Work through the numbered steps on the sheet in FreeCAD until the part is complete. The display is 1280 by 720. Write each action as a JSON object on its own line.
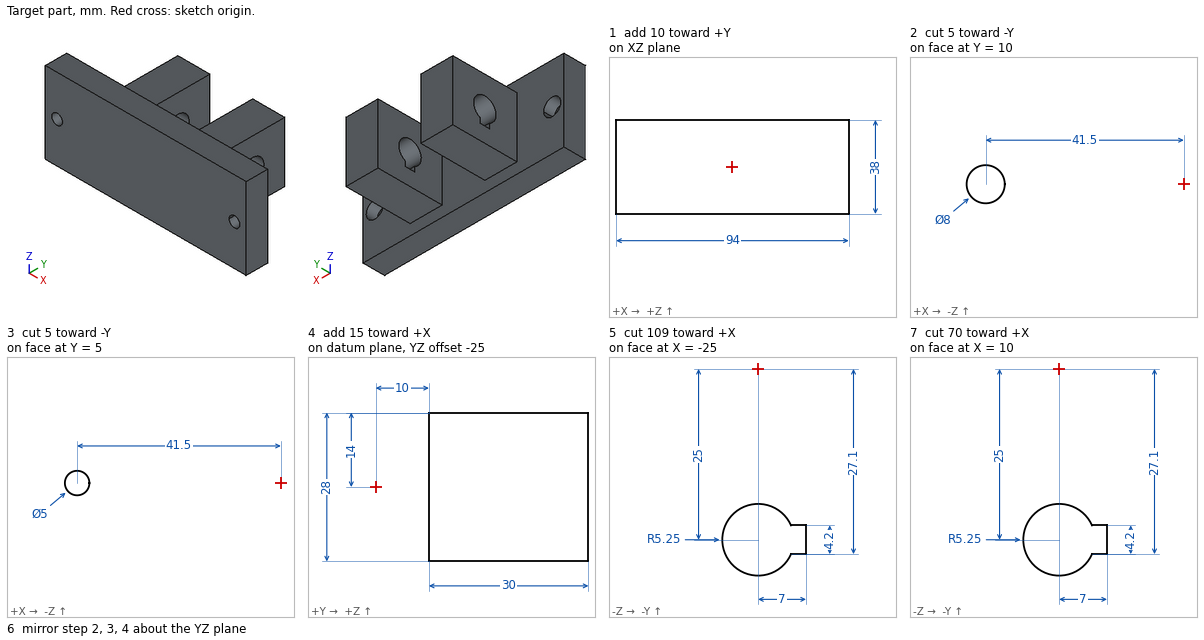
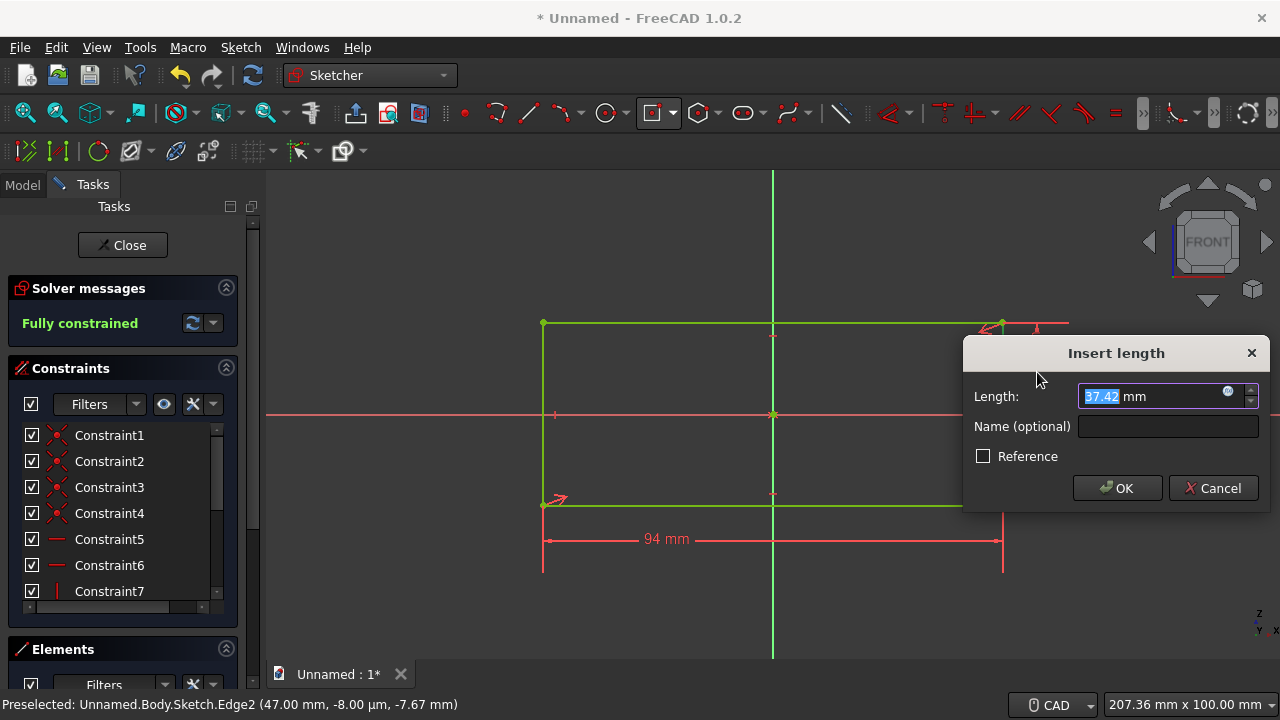
{"action": "type", "text": "38"}
{"action": "key", "text": "Return"}
{"action": "key", "text": "Escape"}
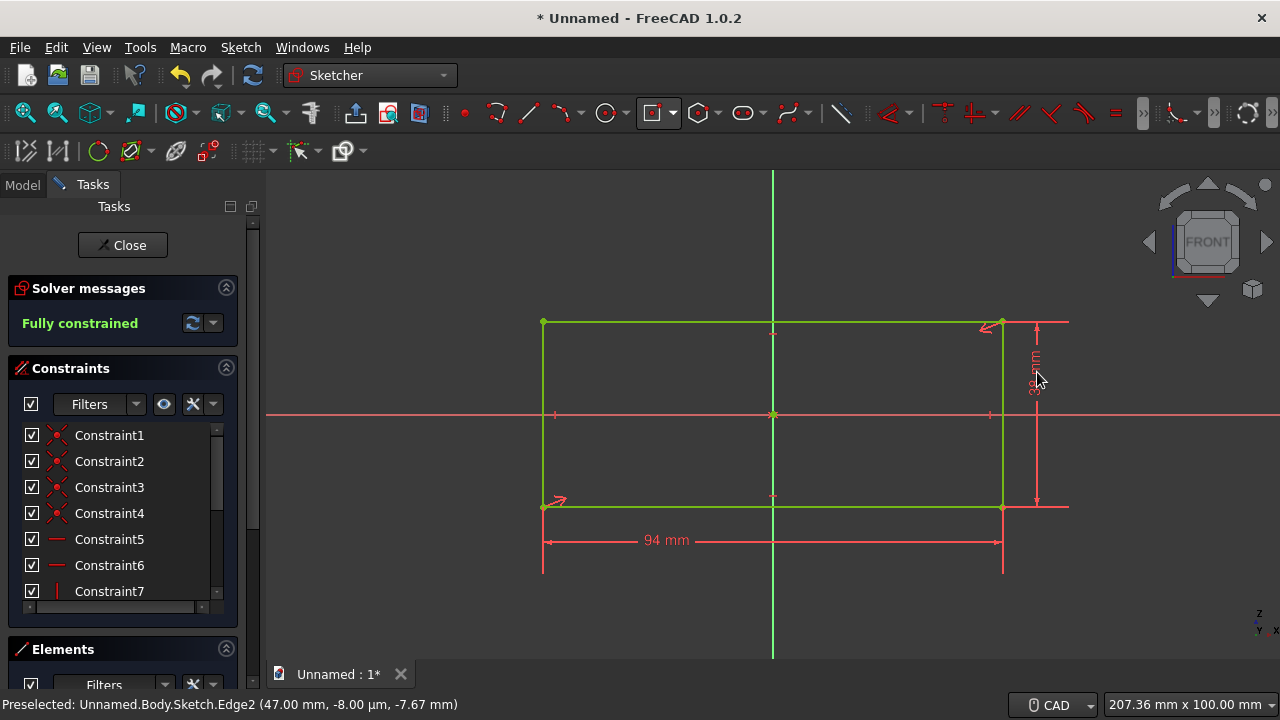
{"action": "left_click", "coordinate": [123, 245]}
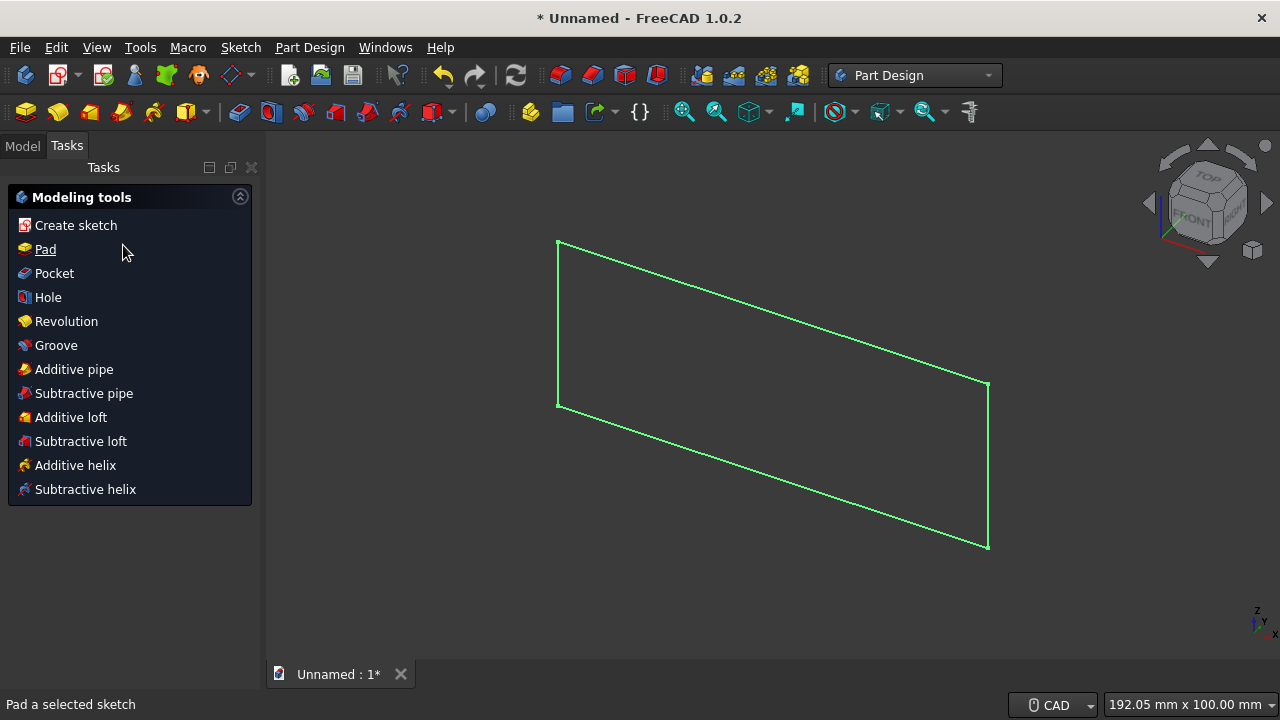
{"action": "left_click", "coordinate": [26, 112]}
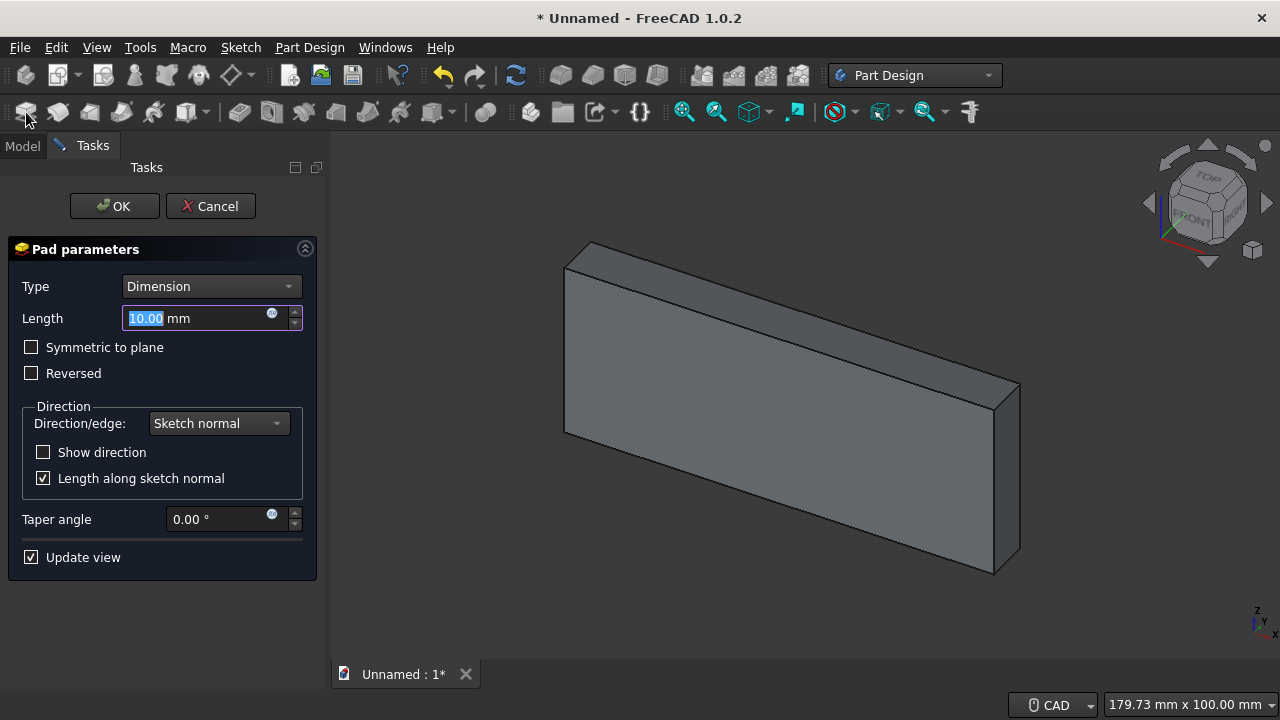
{"action": "type", "text": "10"}
{"action": "key", "text": "Tab"}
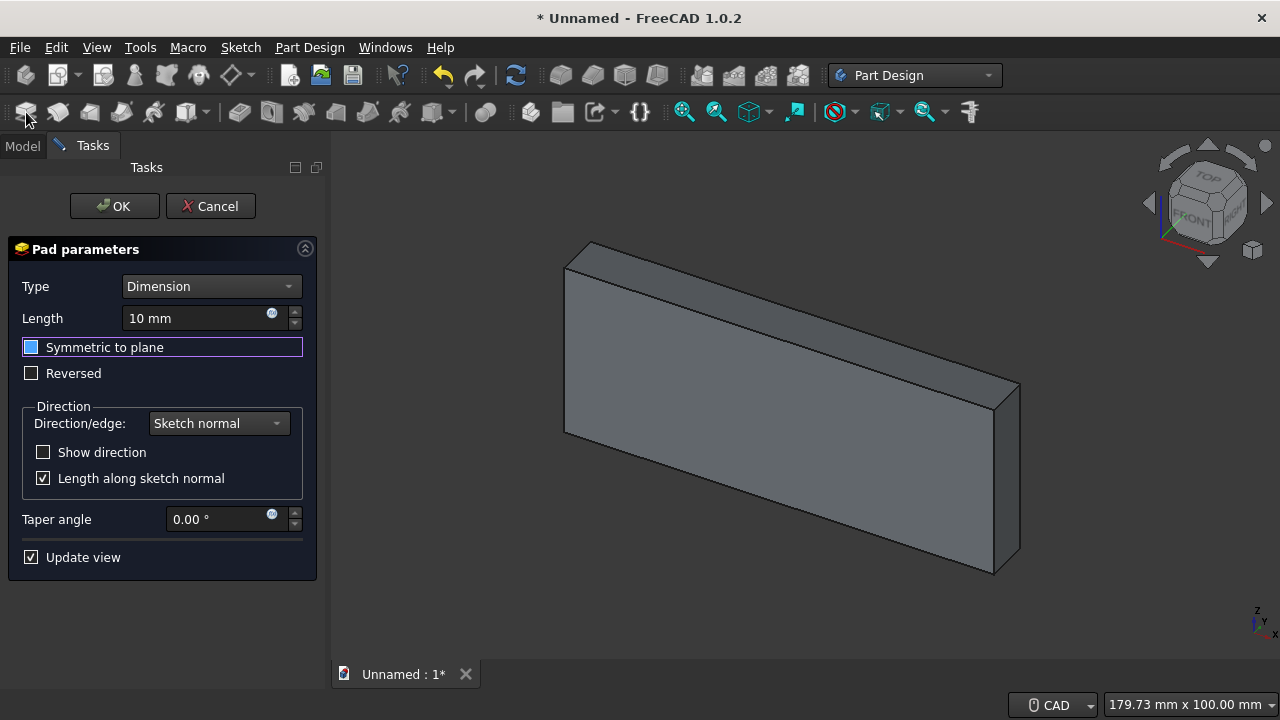
{"action": "left_click", "coordinate": [30, 373]}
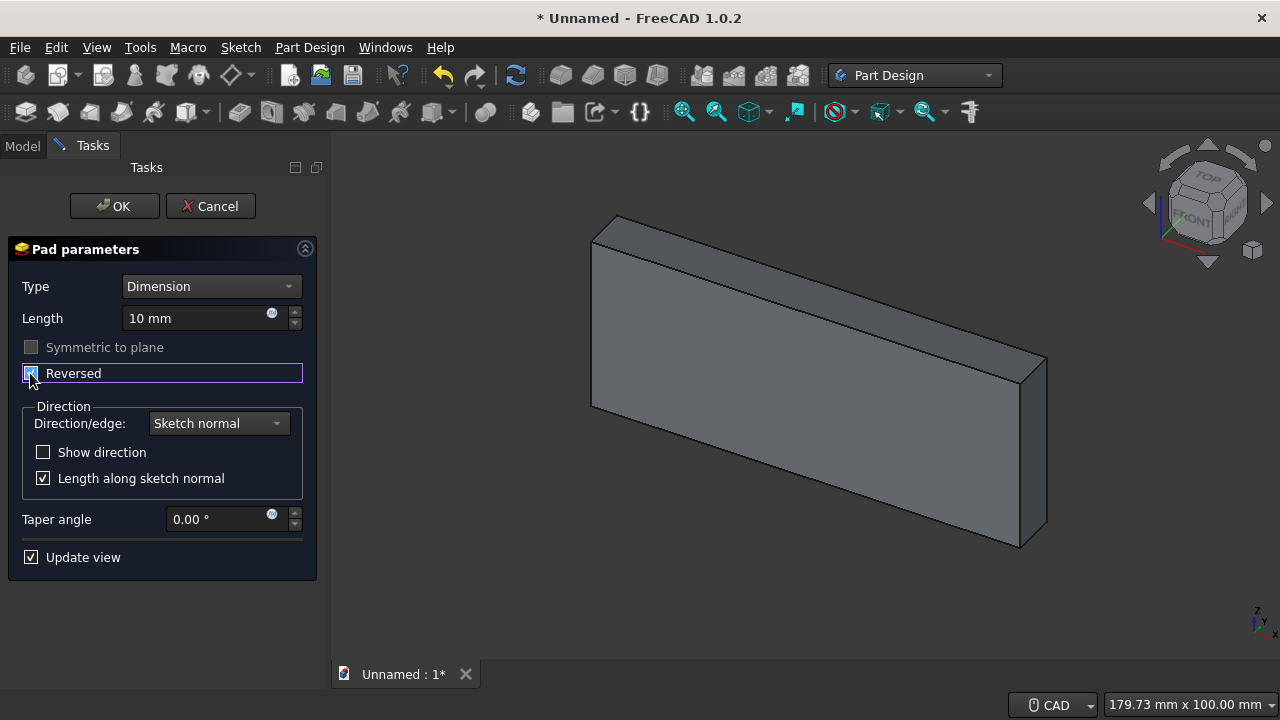
{"action": "left_click", "coordinate": [115, 206]}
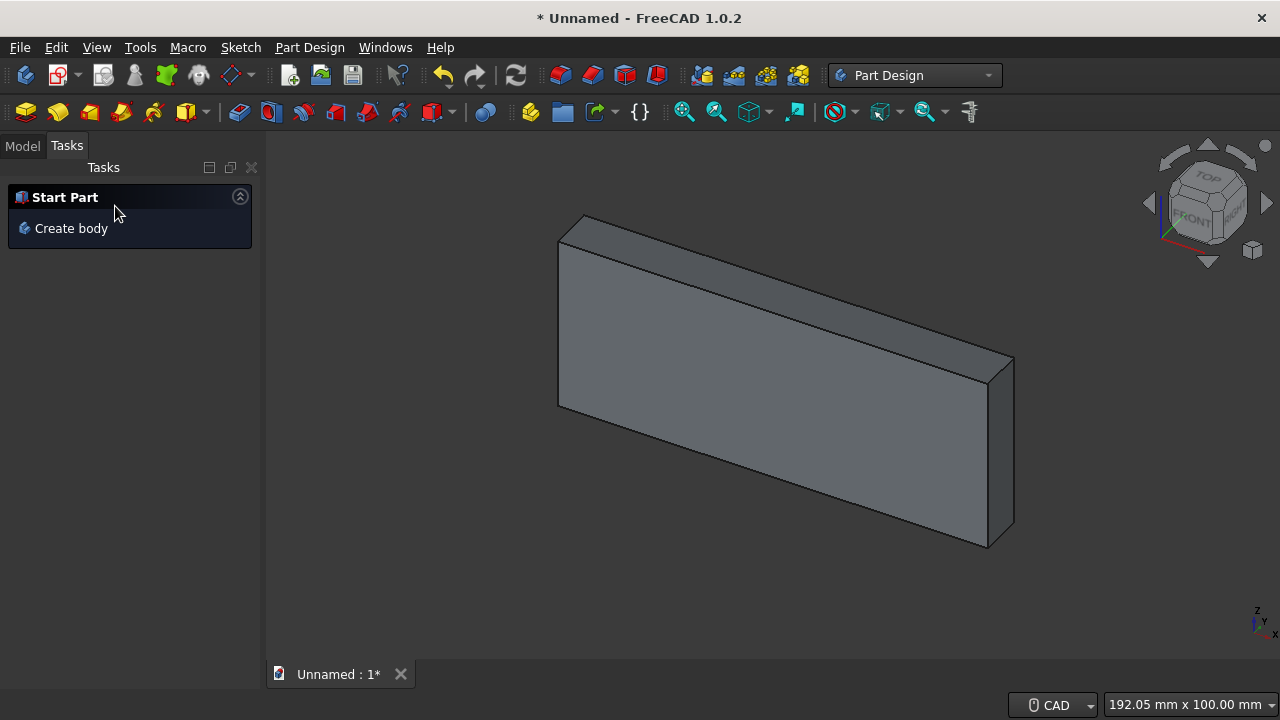
{"action": "key", "text": "4"}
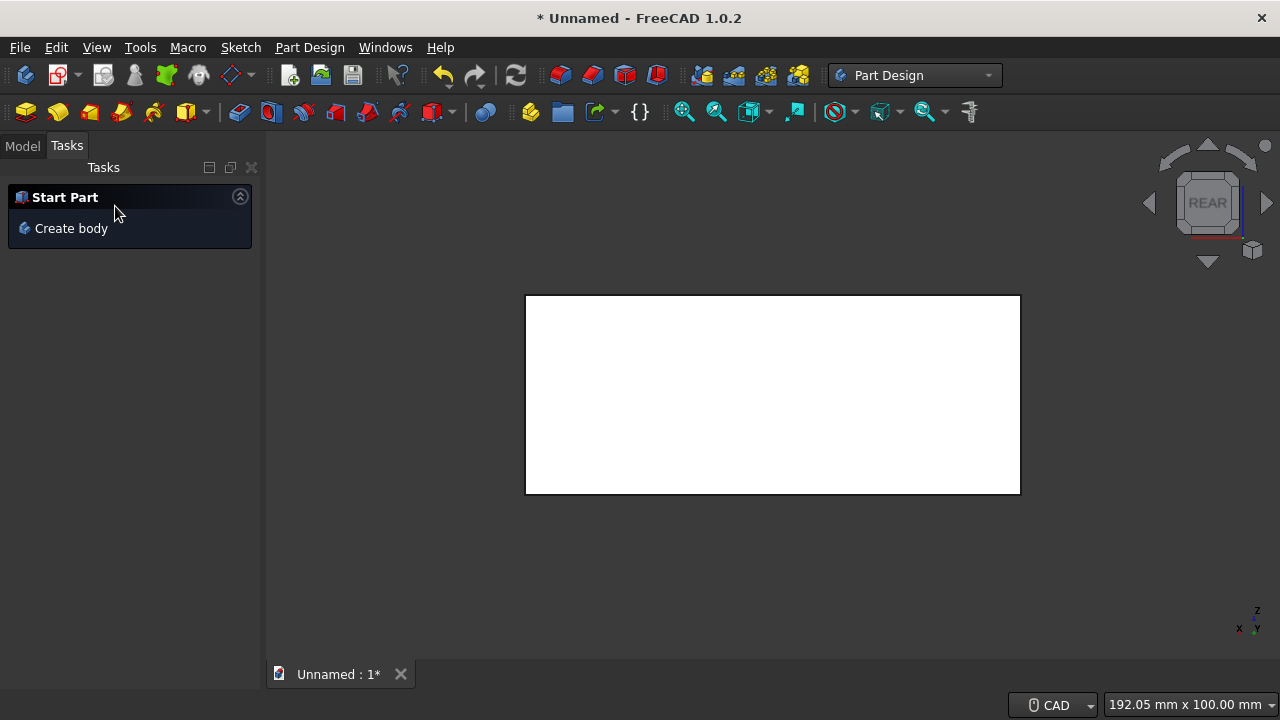
{"action": "left_click", "coordinate": [631, 394]}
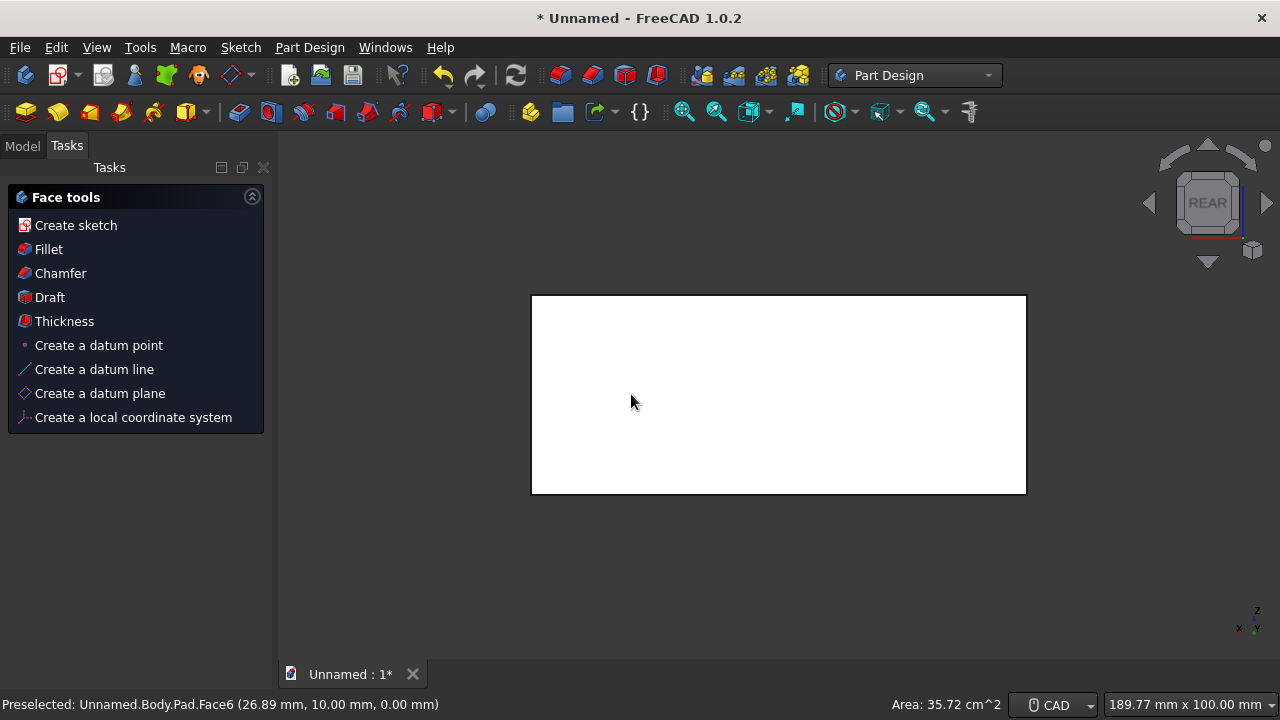
{"action": "left_click", "coordinate": [58, 76]}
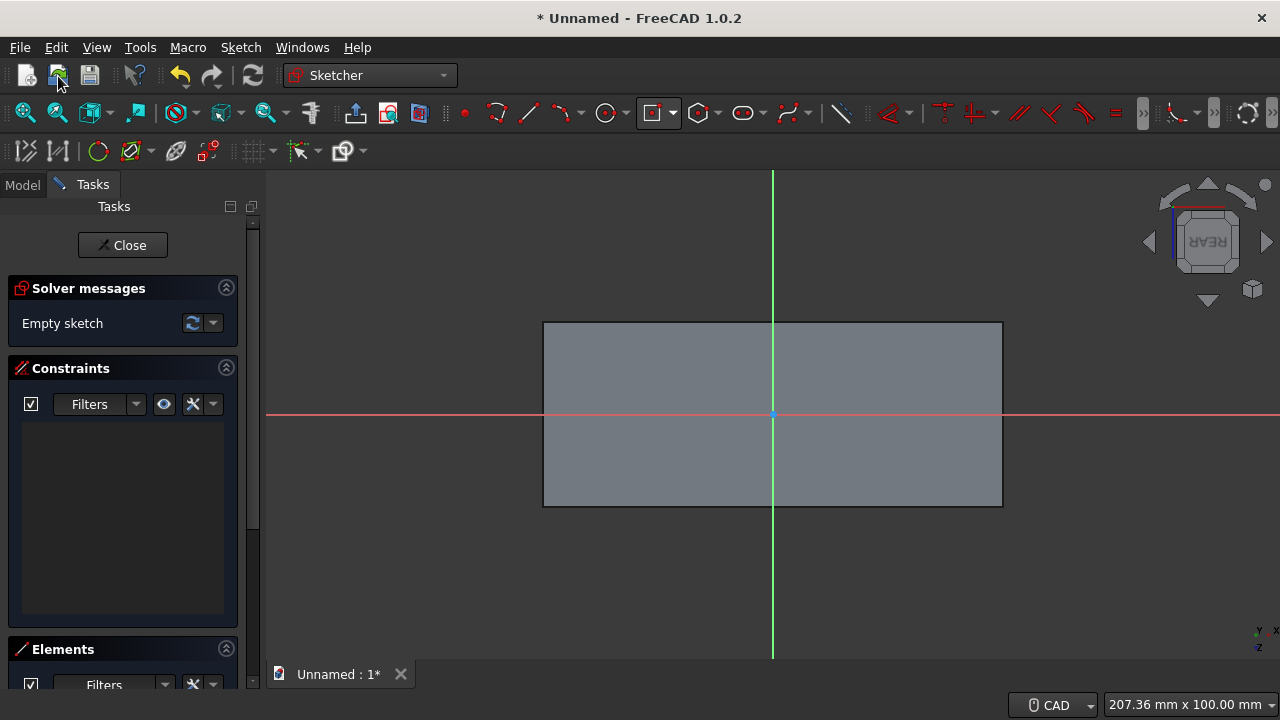
{"action": "scroll", "coordinate": [549, 415], "scroll_direction": "up", "scroll_amount": 10}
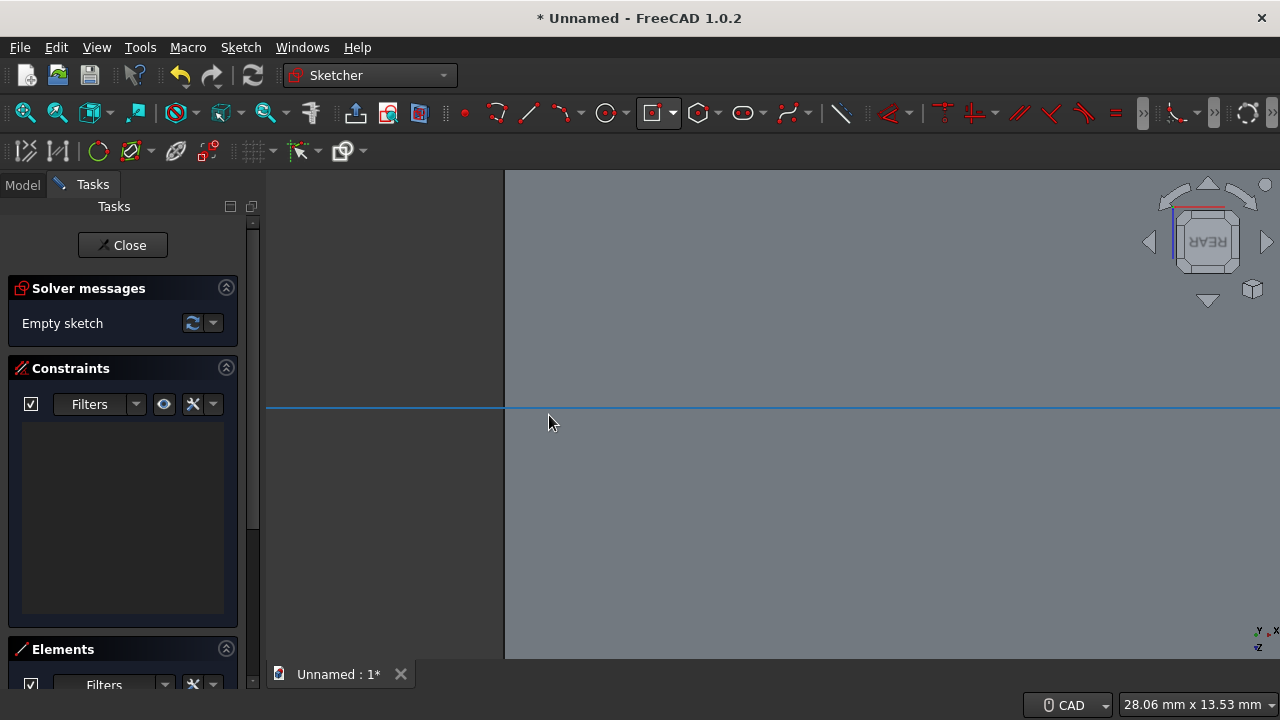
{"action": "left_click", "coordinate": [606, 114]}